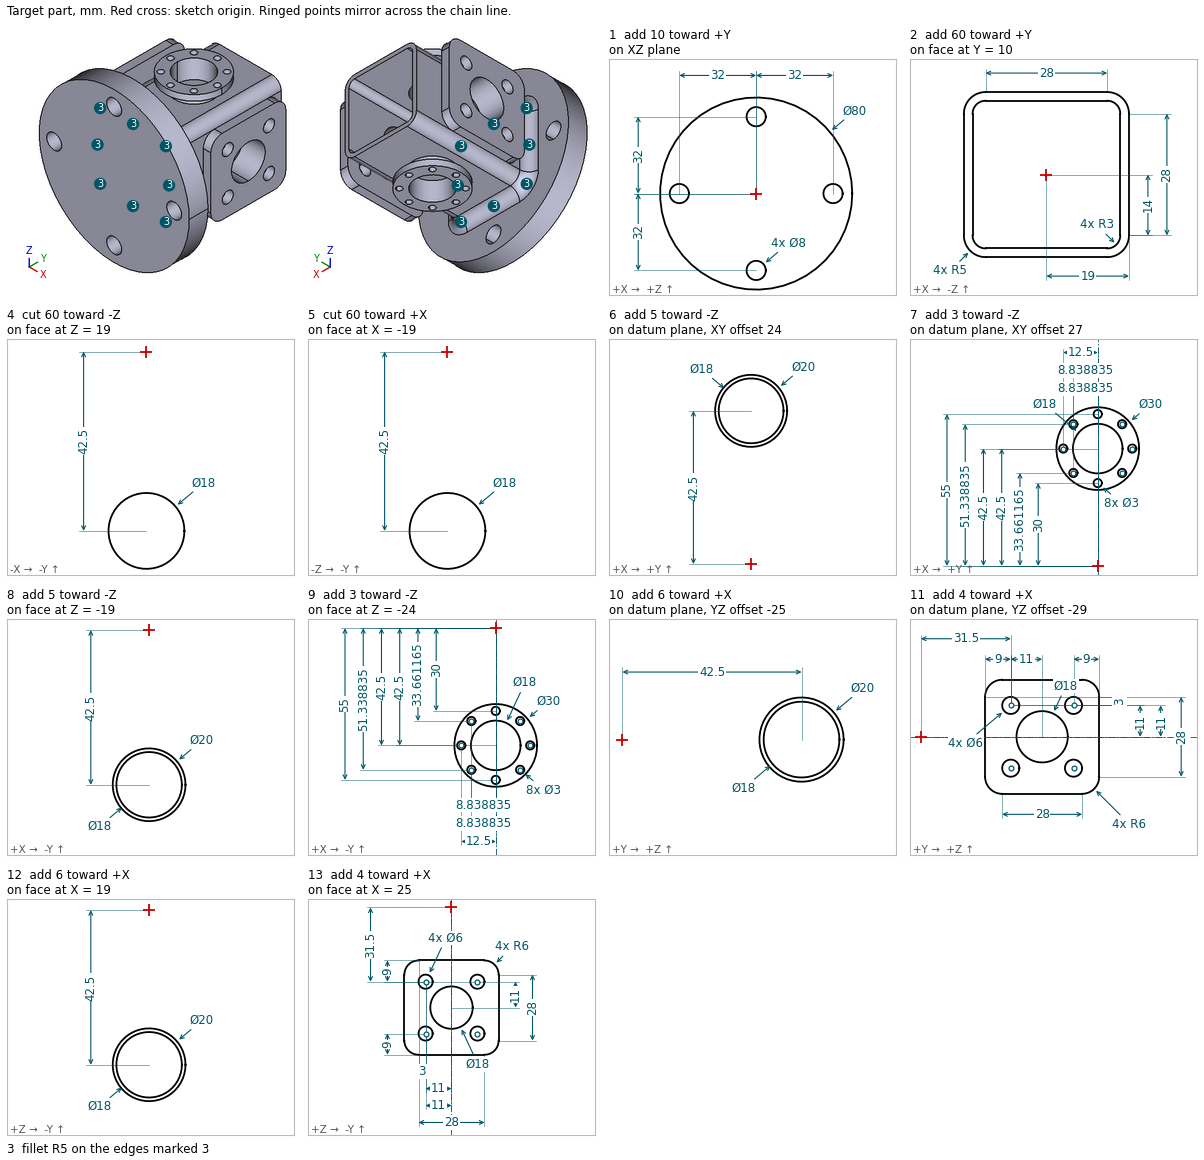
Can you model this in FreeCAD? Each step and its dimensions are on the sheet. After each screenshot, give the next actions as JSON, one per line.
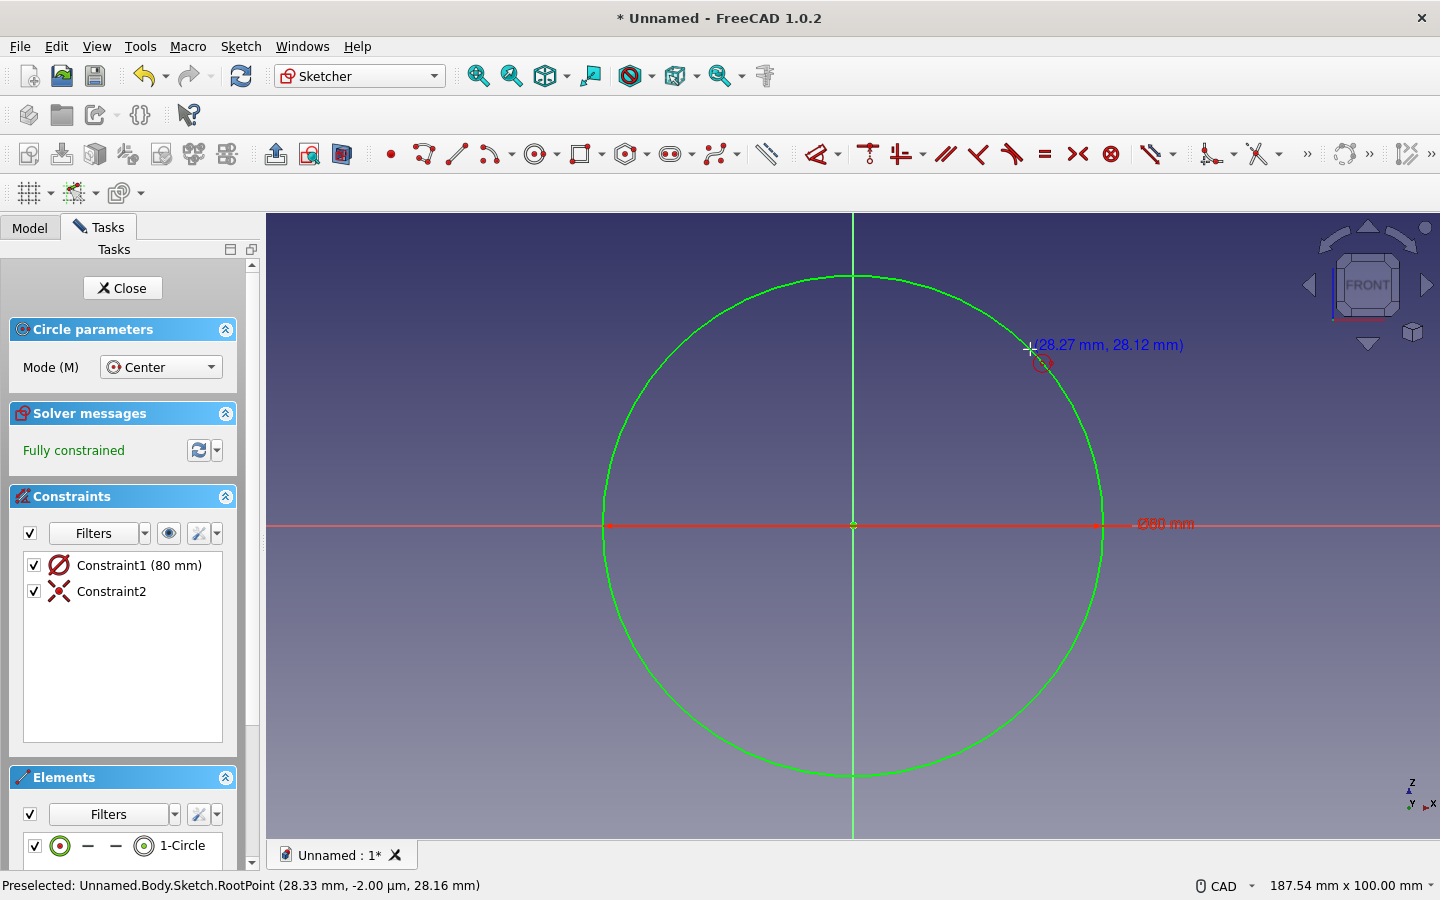
{"action": "left_click", "coordinate": [853, 726]}
{"action": "mouse_move", "coordinate": [871, 709]}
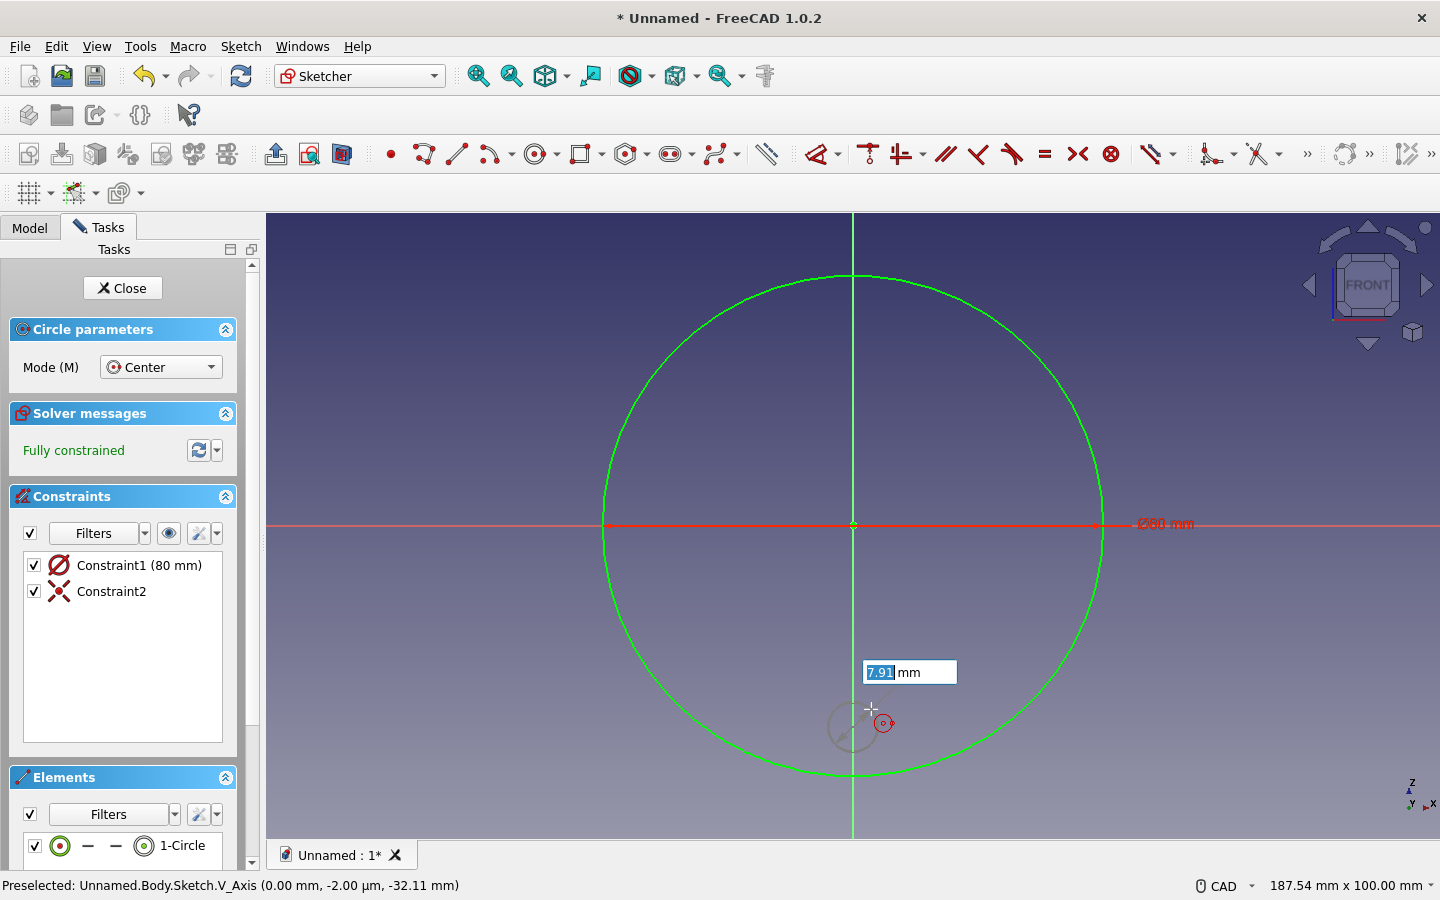
{"action": "type", "text": "8"}
{"action": "key", "text": "Return"}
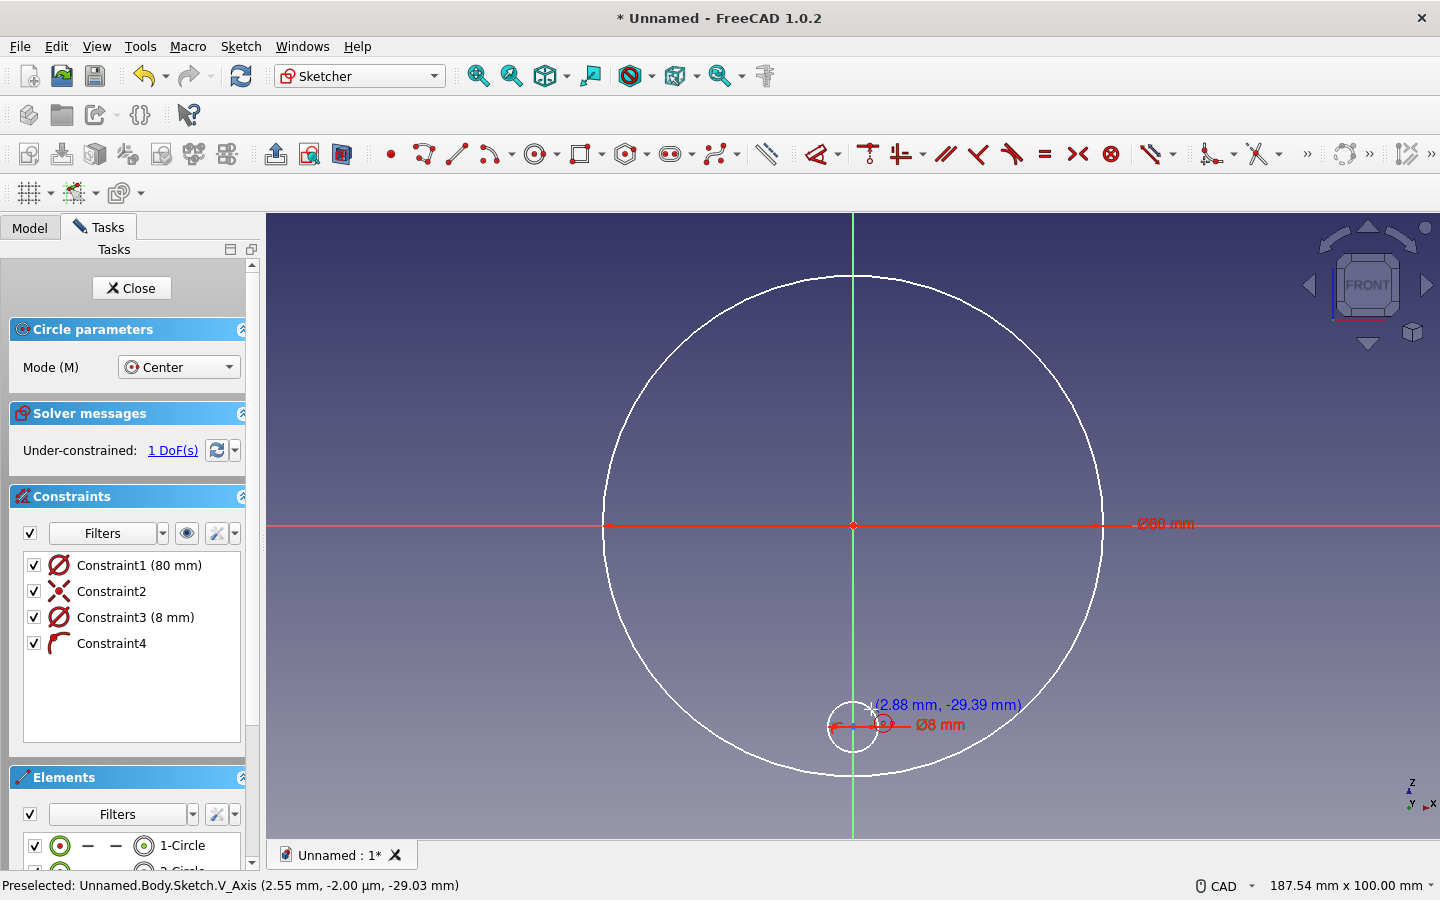
{"action": "left_click", "coordinate": [653, 526]}
{"action": "mouse_move", "coordinate": [670, 508]}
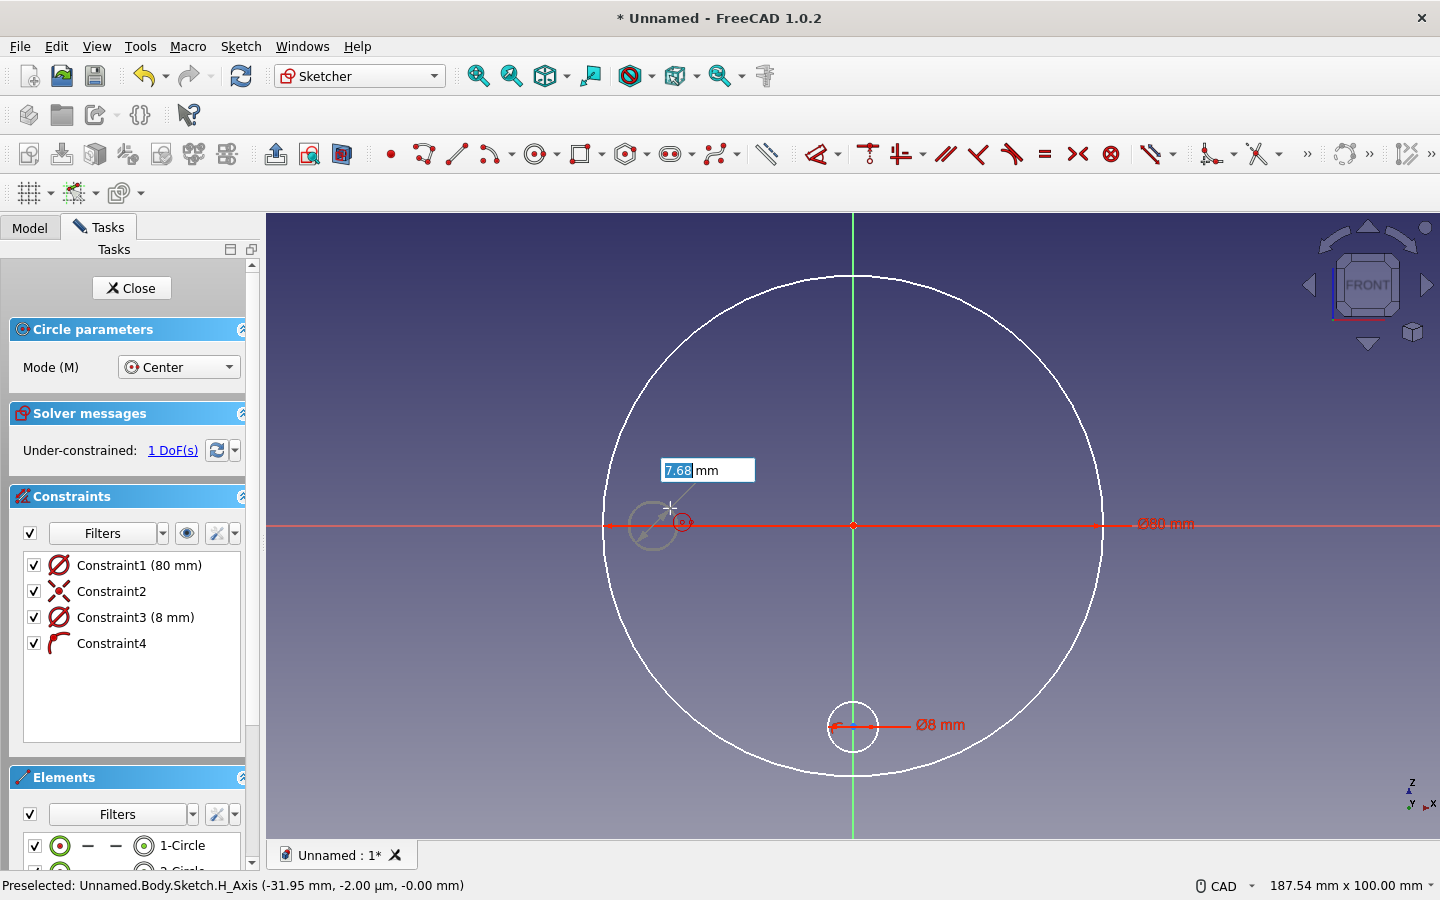
{"action": "type", "text": "8"}
{"action": "key", "text": "Return"}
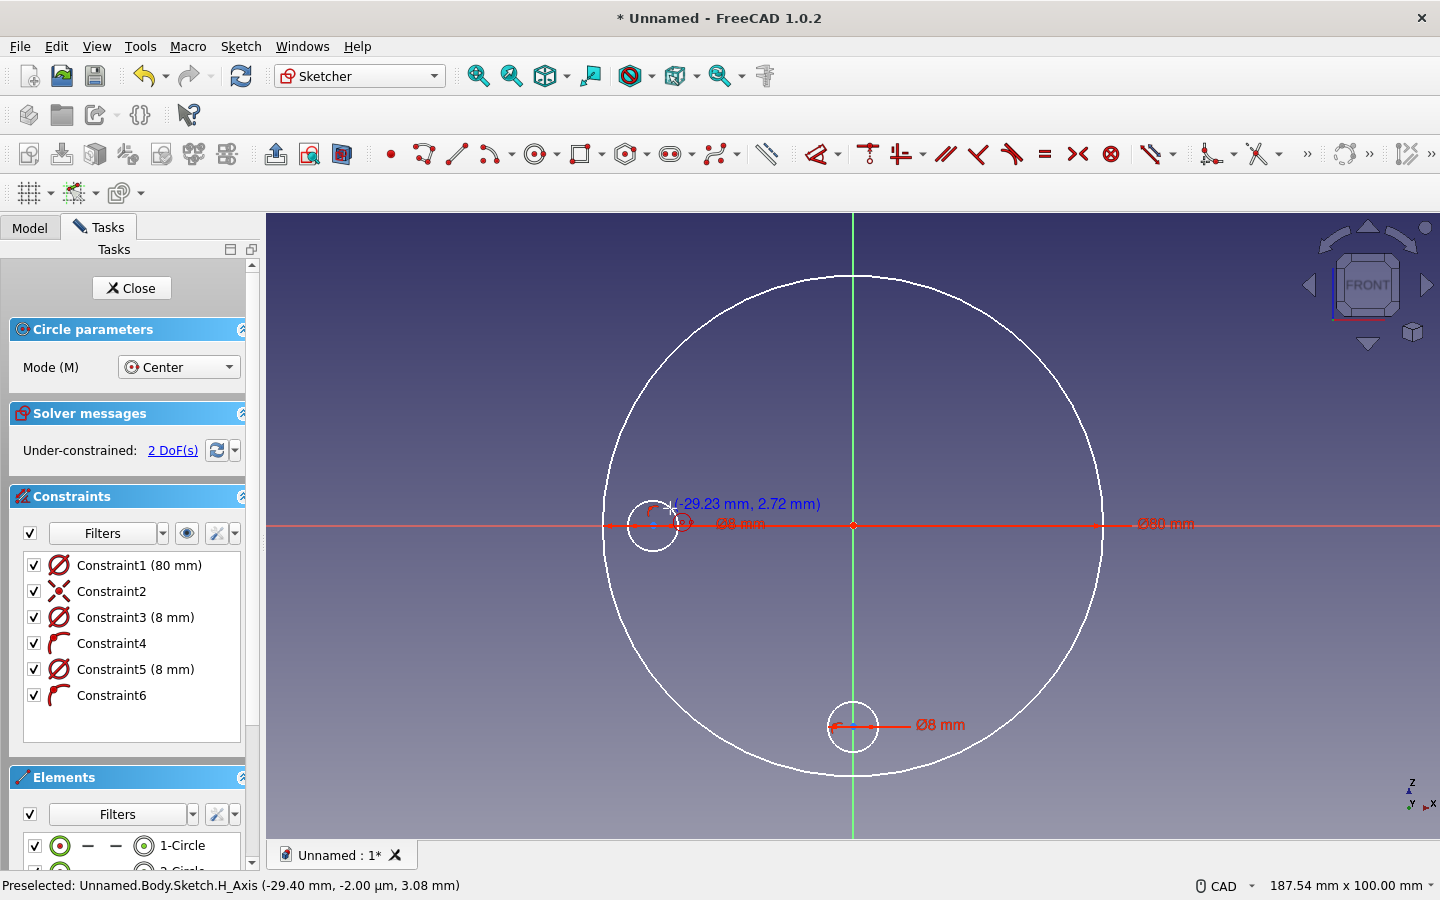
{"action": "left_click", "coordinate": [1053, 526]}
{"action": "mouse_move", "coordinate": [1071, 508]}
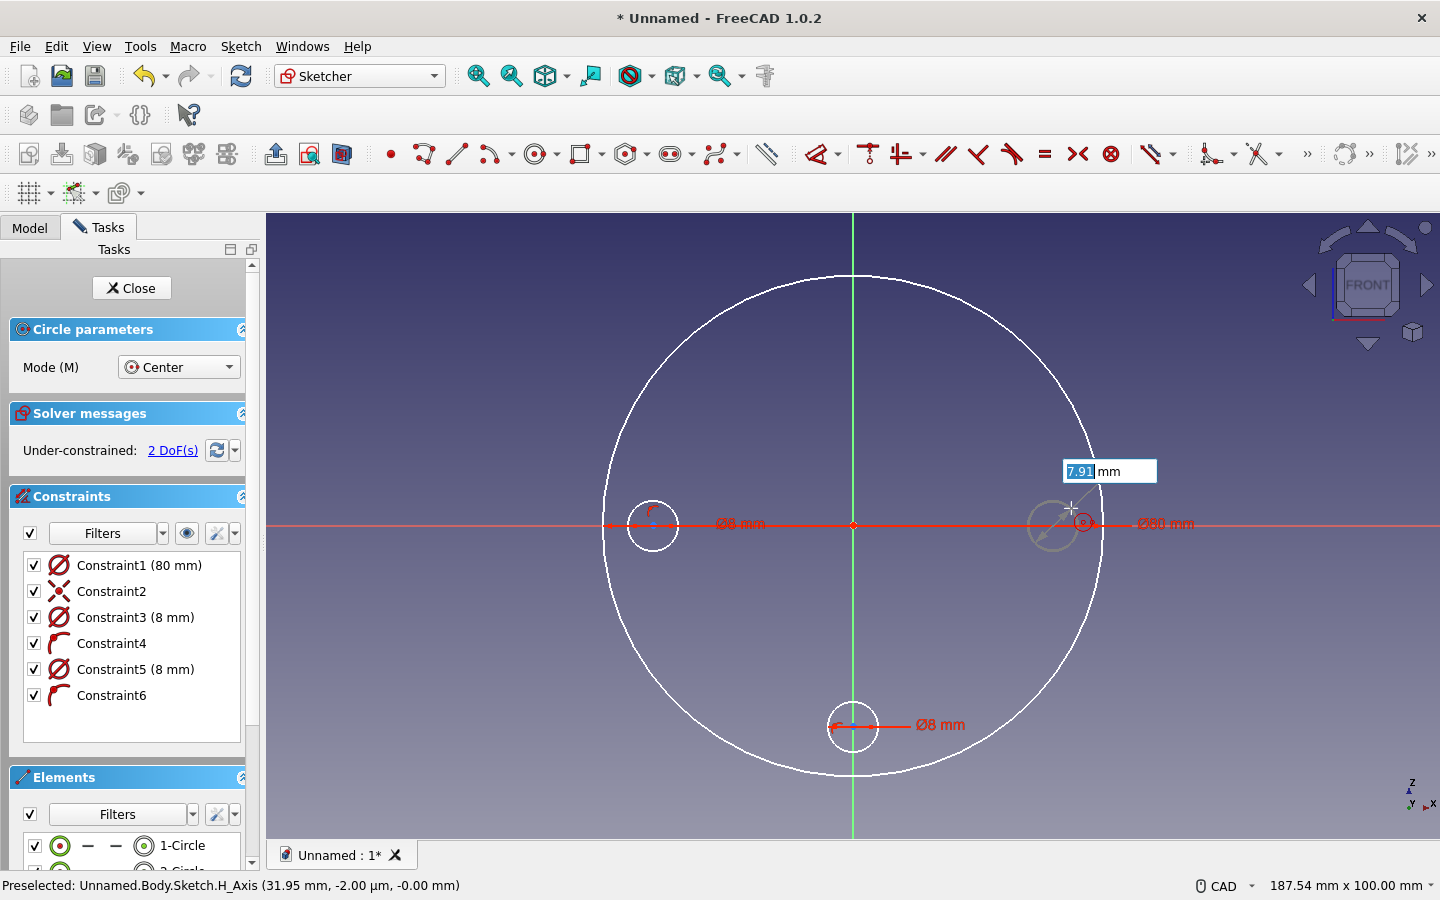
{"action": "type", "text": "8"}
{"action": "key", "text": "Return"}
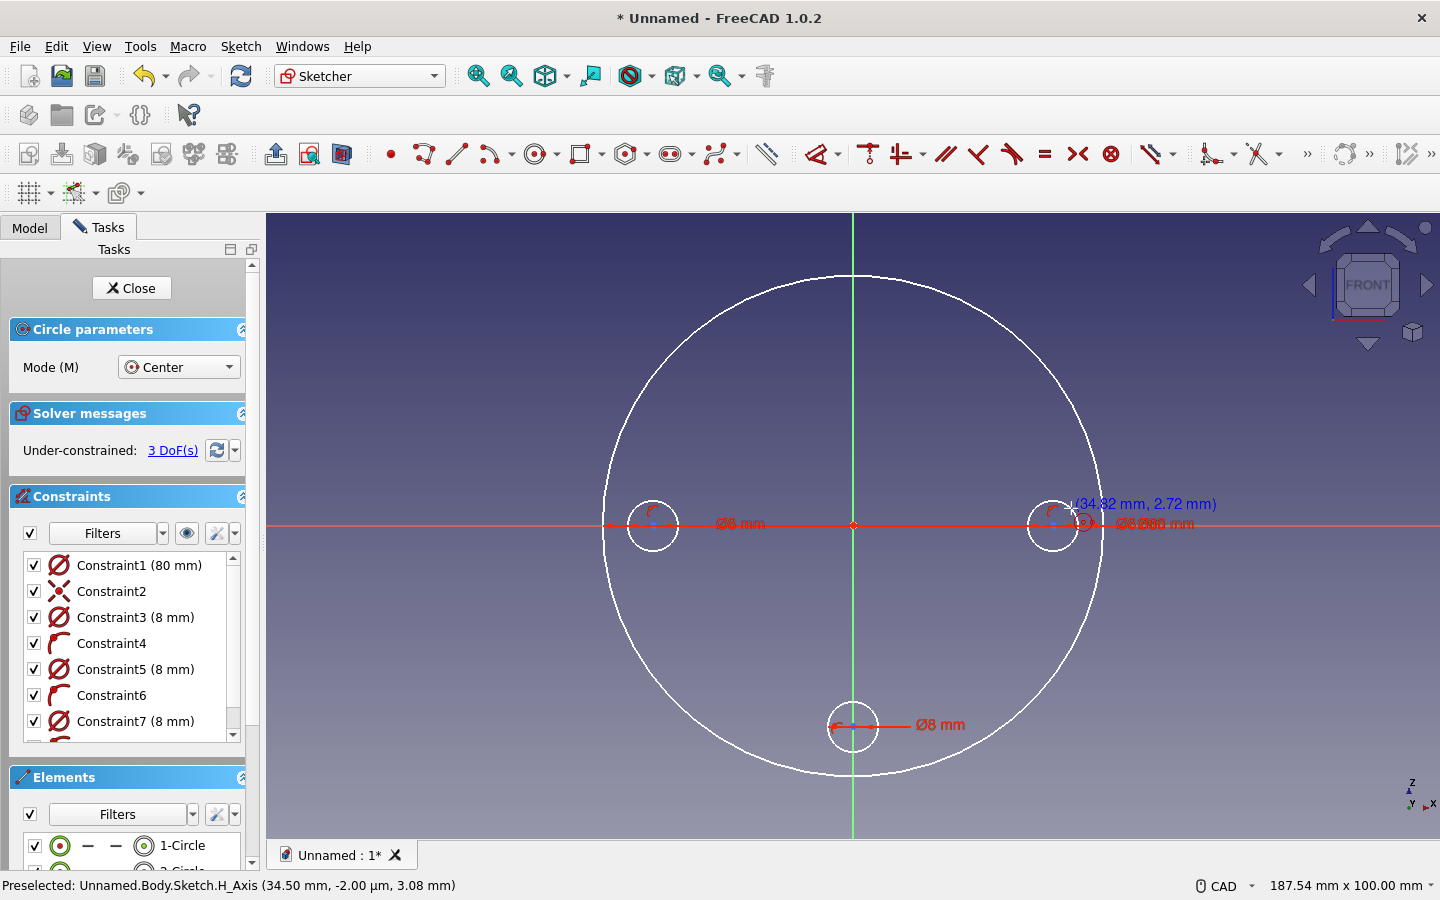
{"action": "left_click", "coordinate": [853, 326]}
{"action": "mouse_move", "coordinate": [871, 308]}